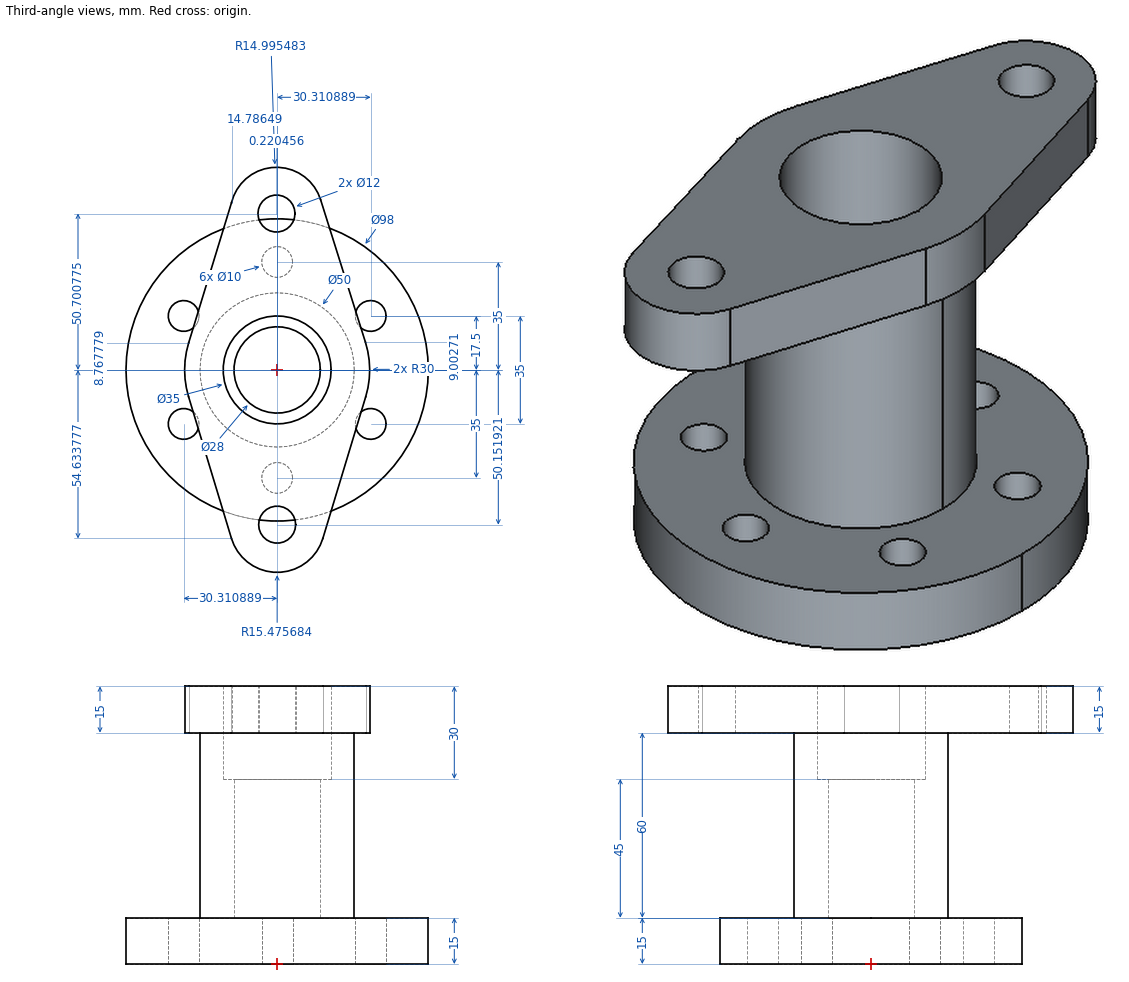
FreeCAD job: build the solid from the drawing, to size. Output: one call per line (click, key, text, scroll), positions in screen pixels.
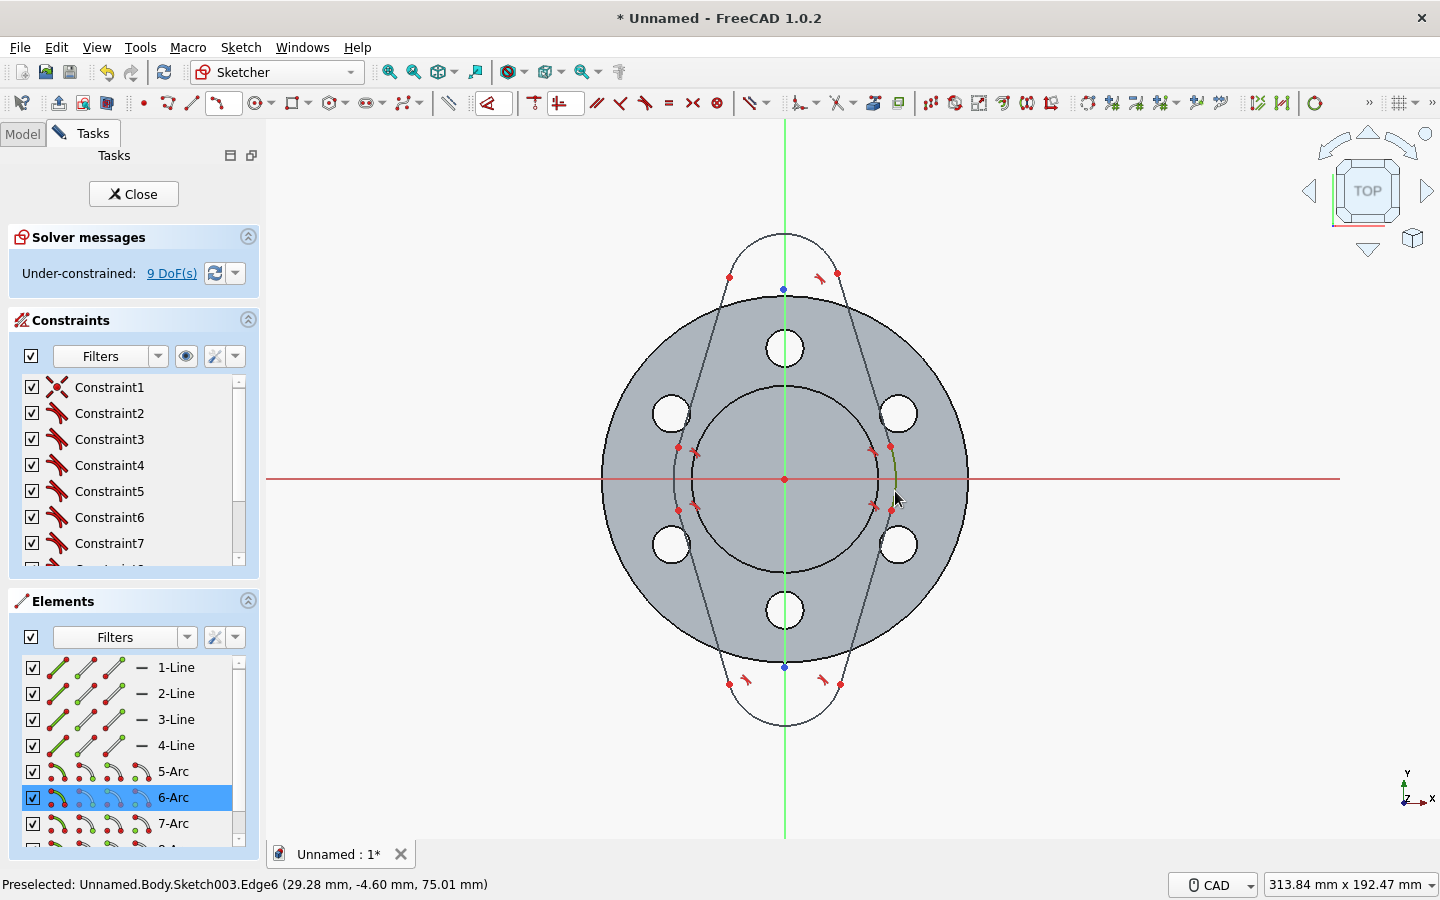
click(674, 466)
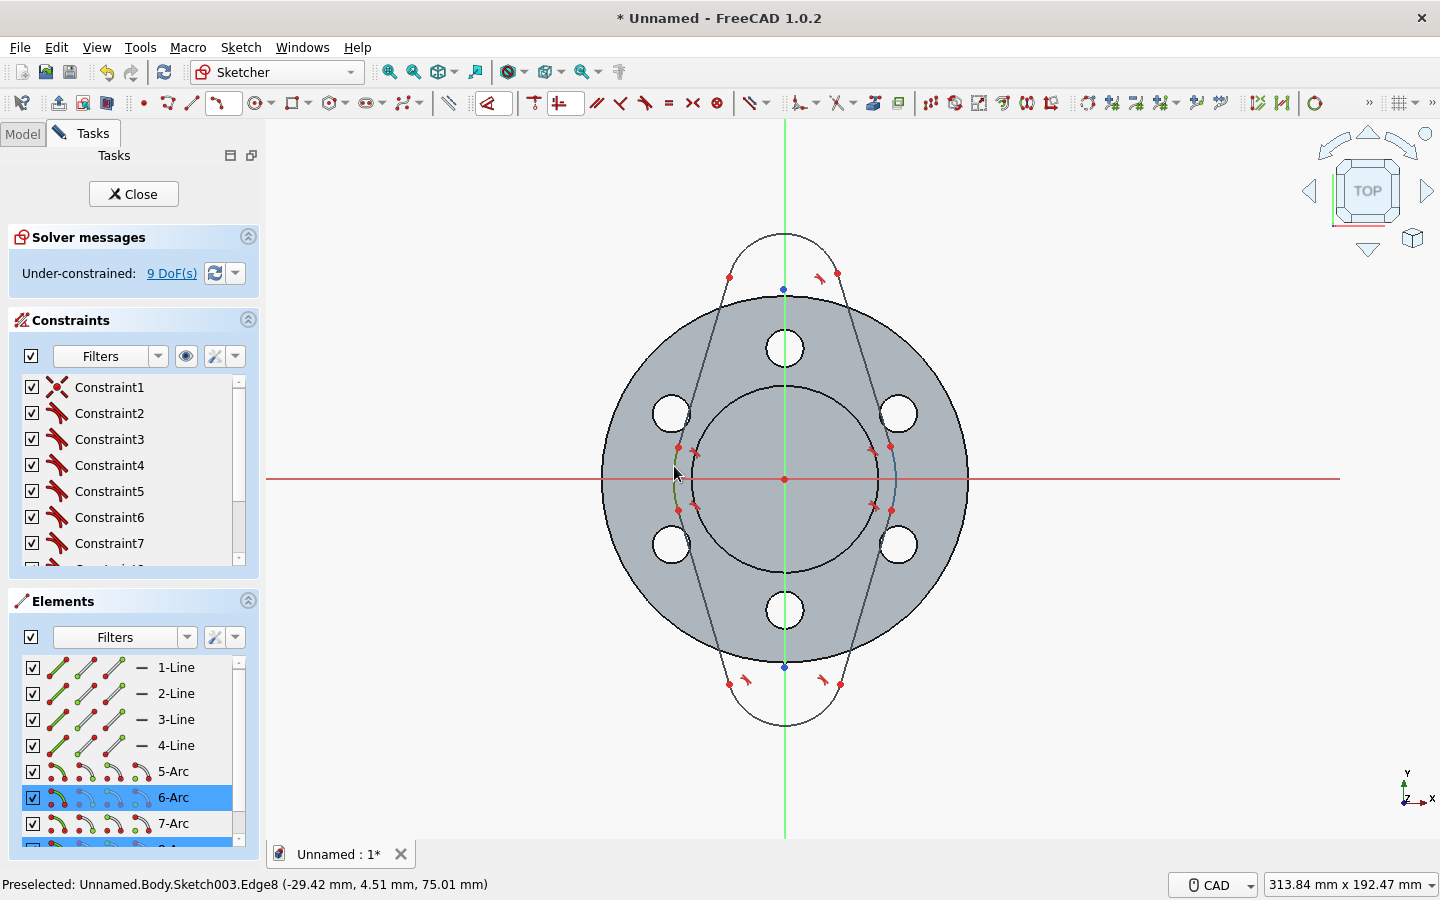
key(e)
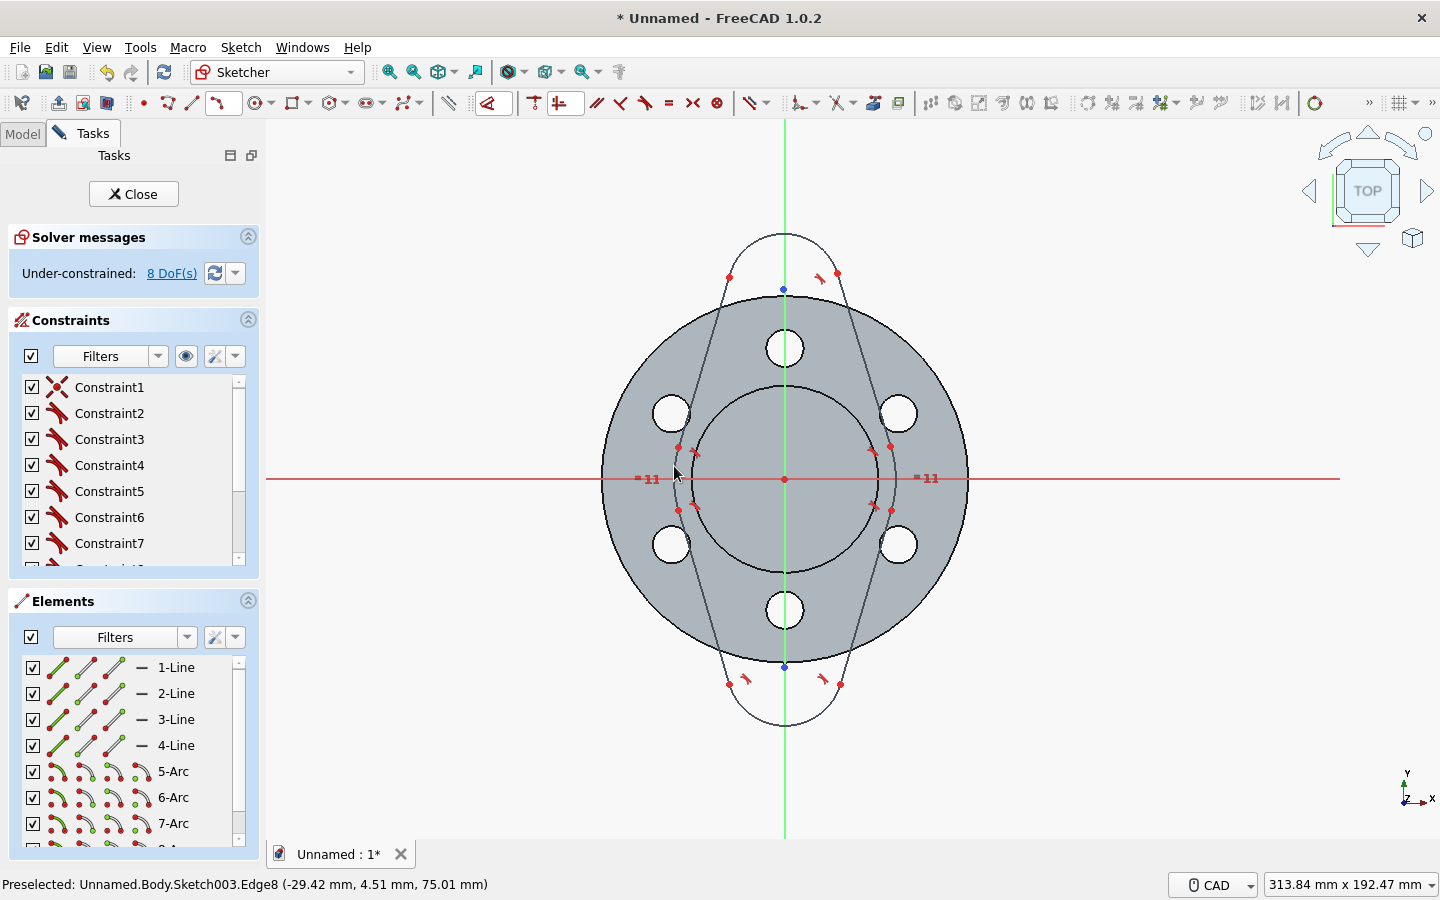
click(785, 668)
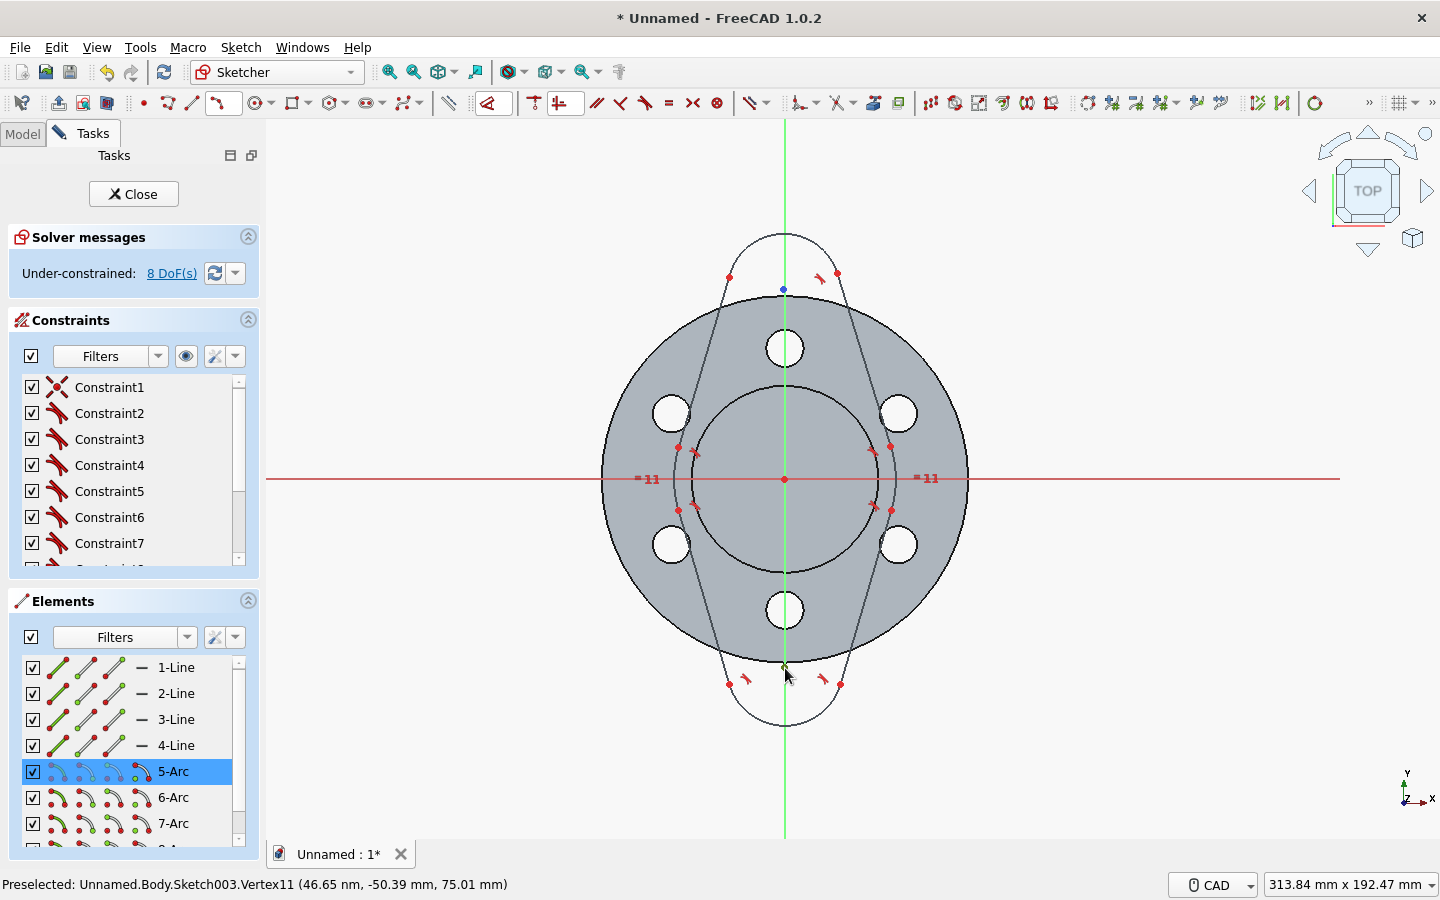
click(785, 764)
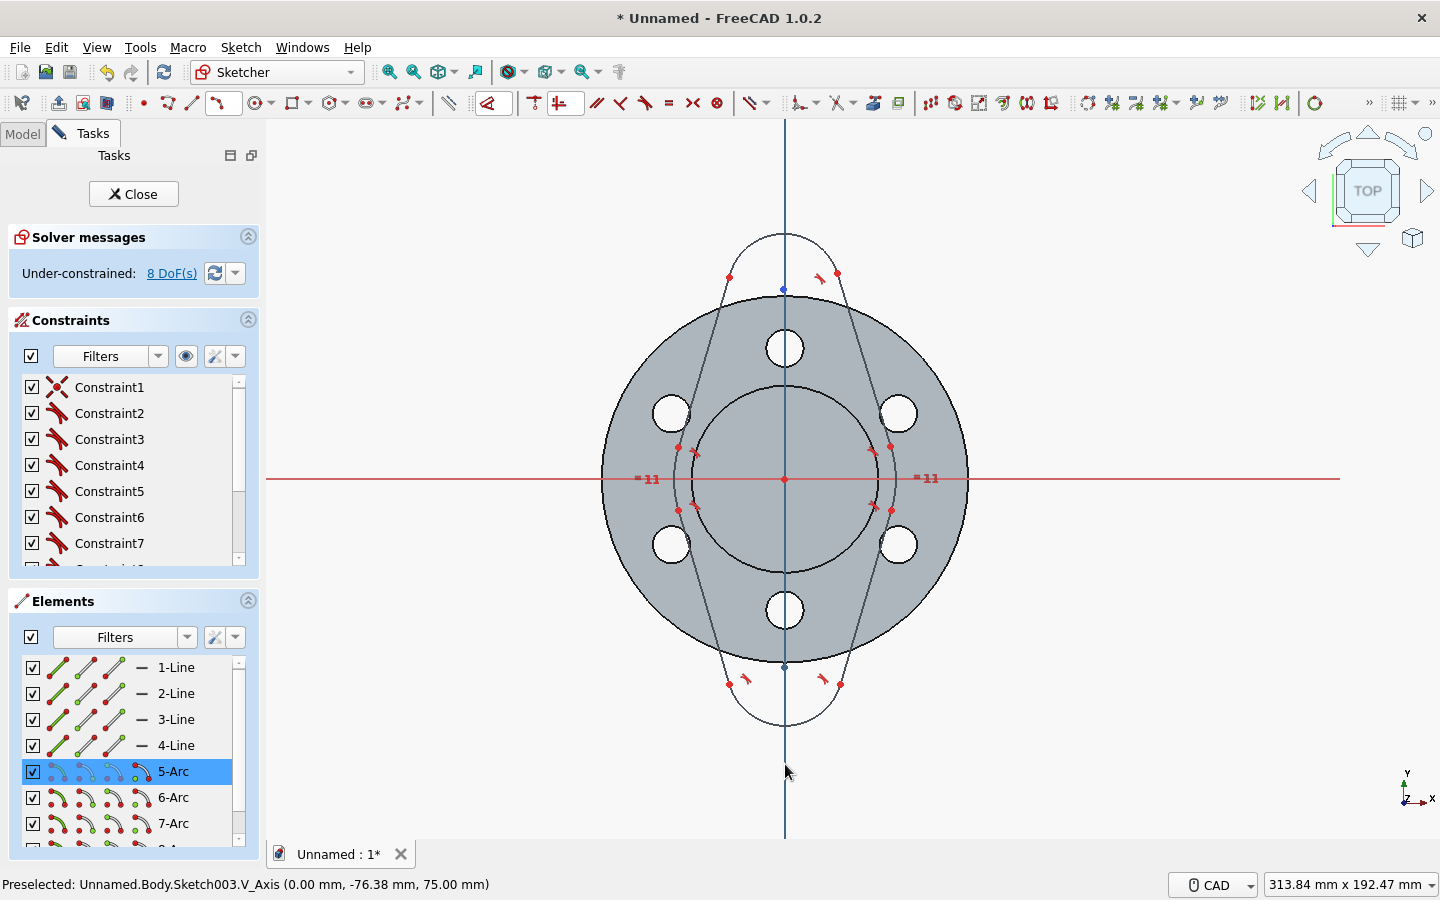
key(c)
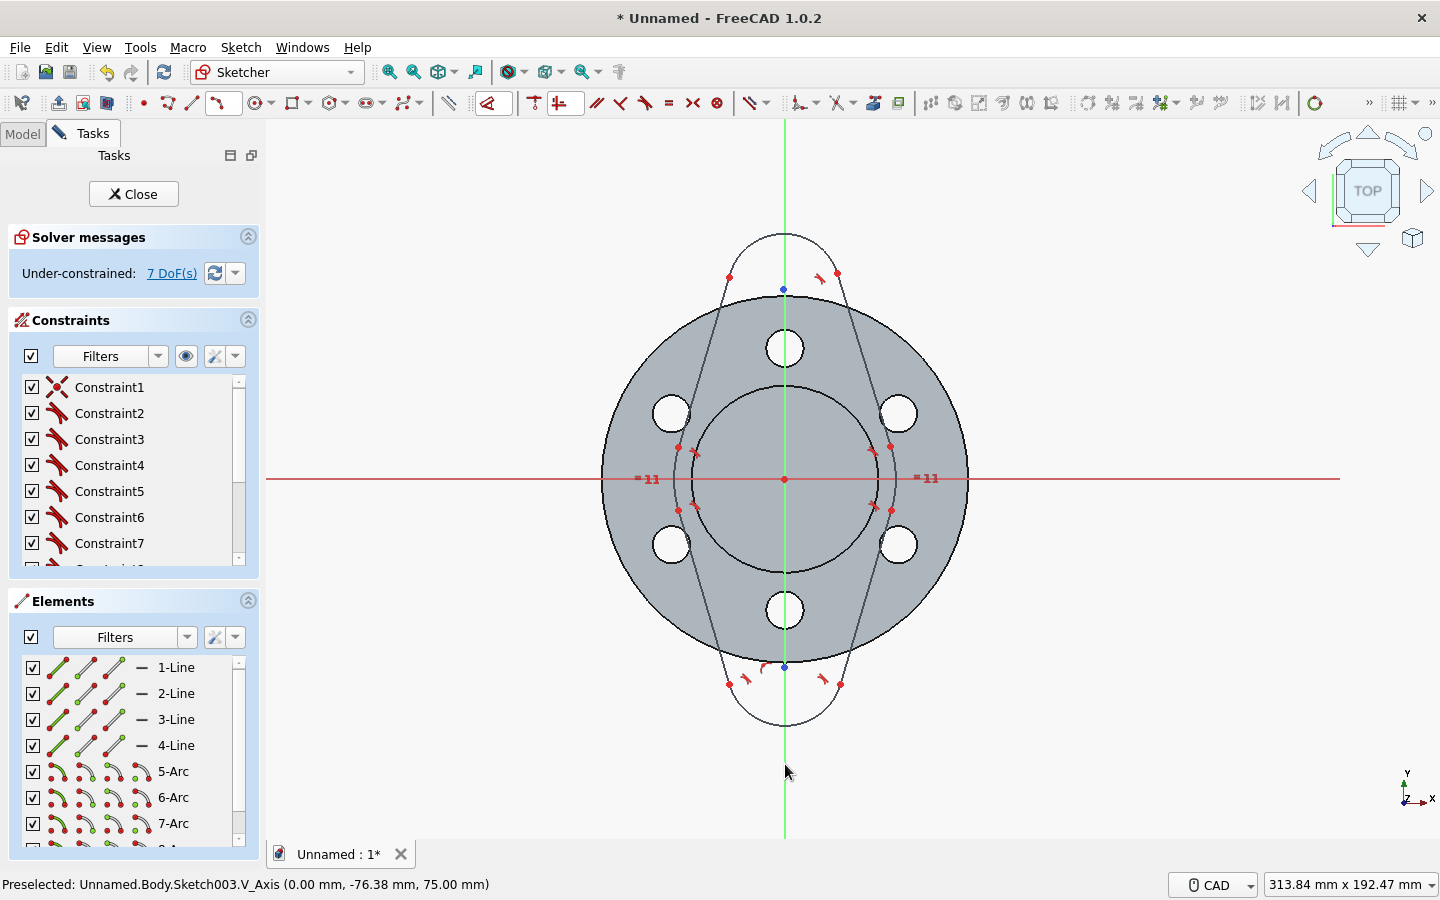
click(756, 718)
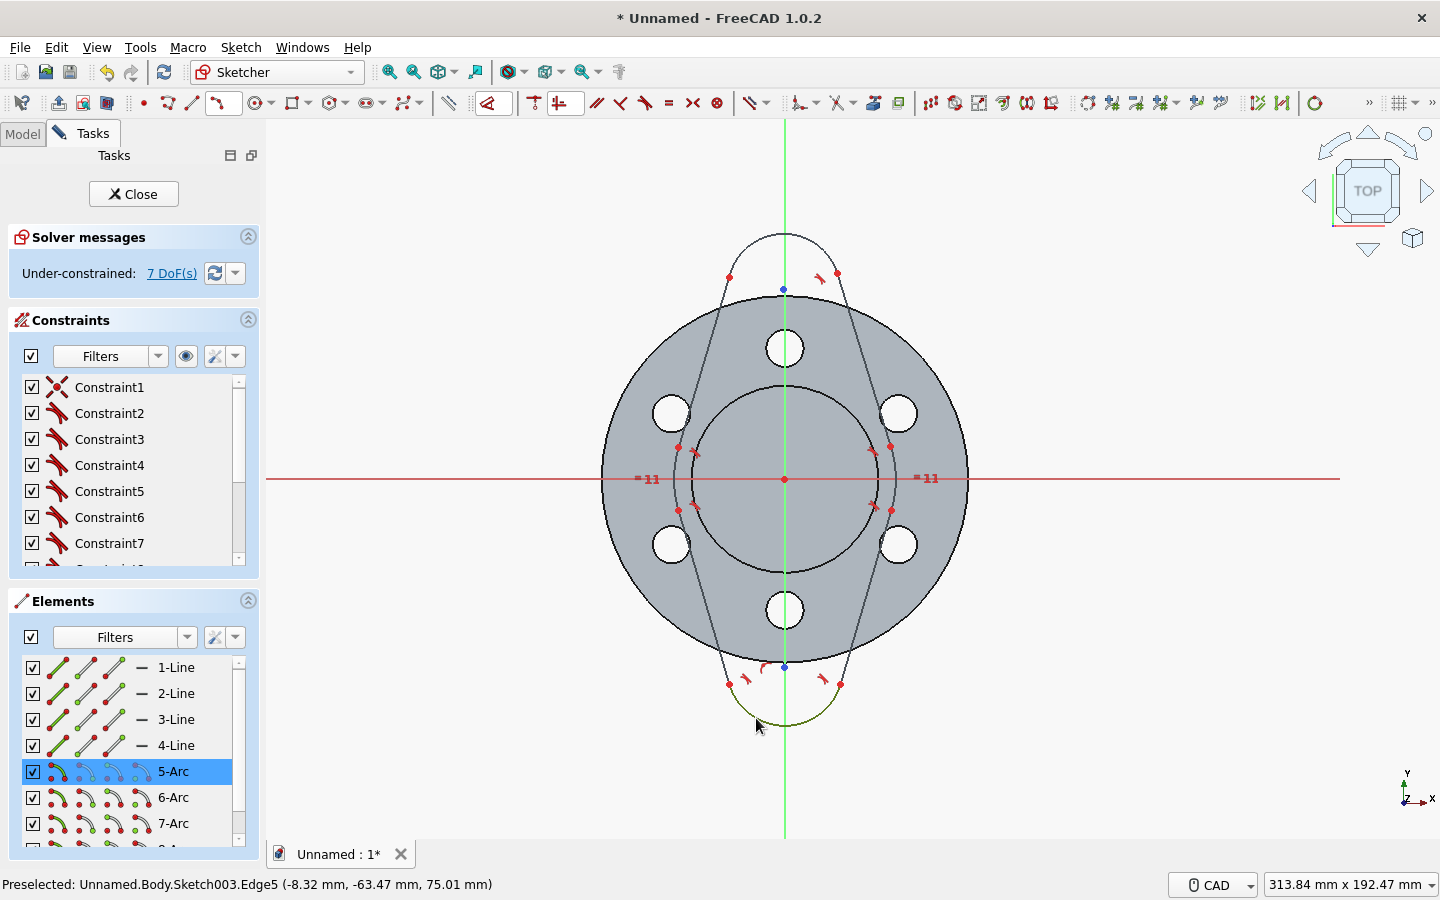
key(k)
key(r)